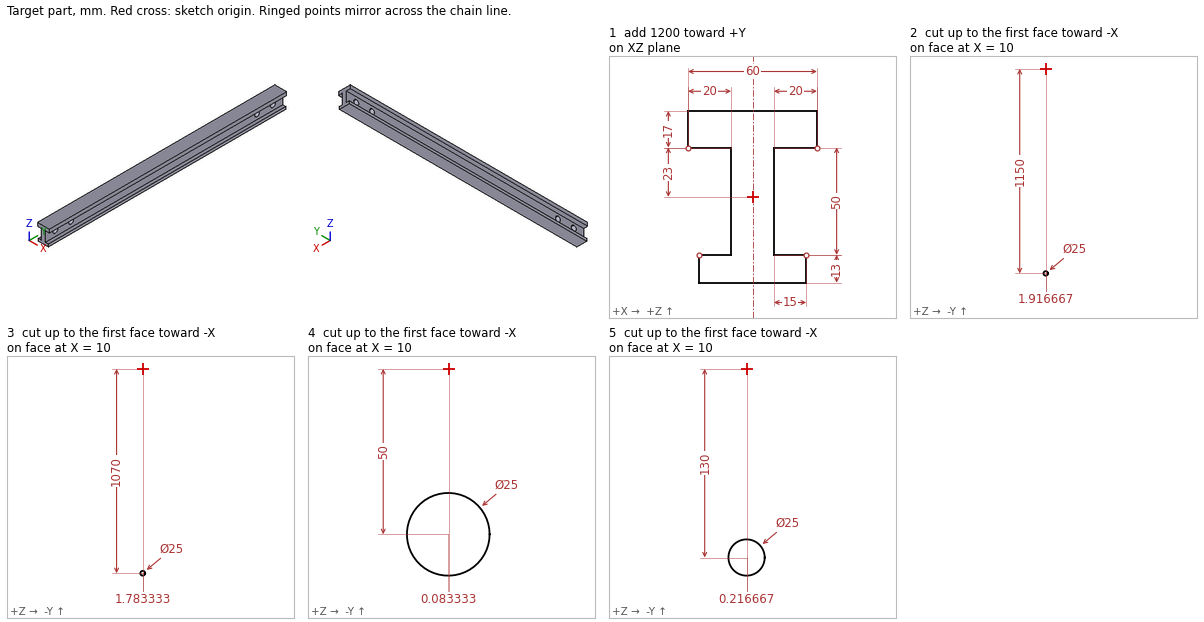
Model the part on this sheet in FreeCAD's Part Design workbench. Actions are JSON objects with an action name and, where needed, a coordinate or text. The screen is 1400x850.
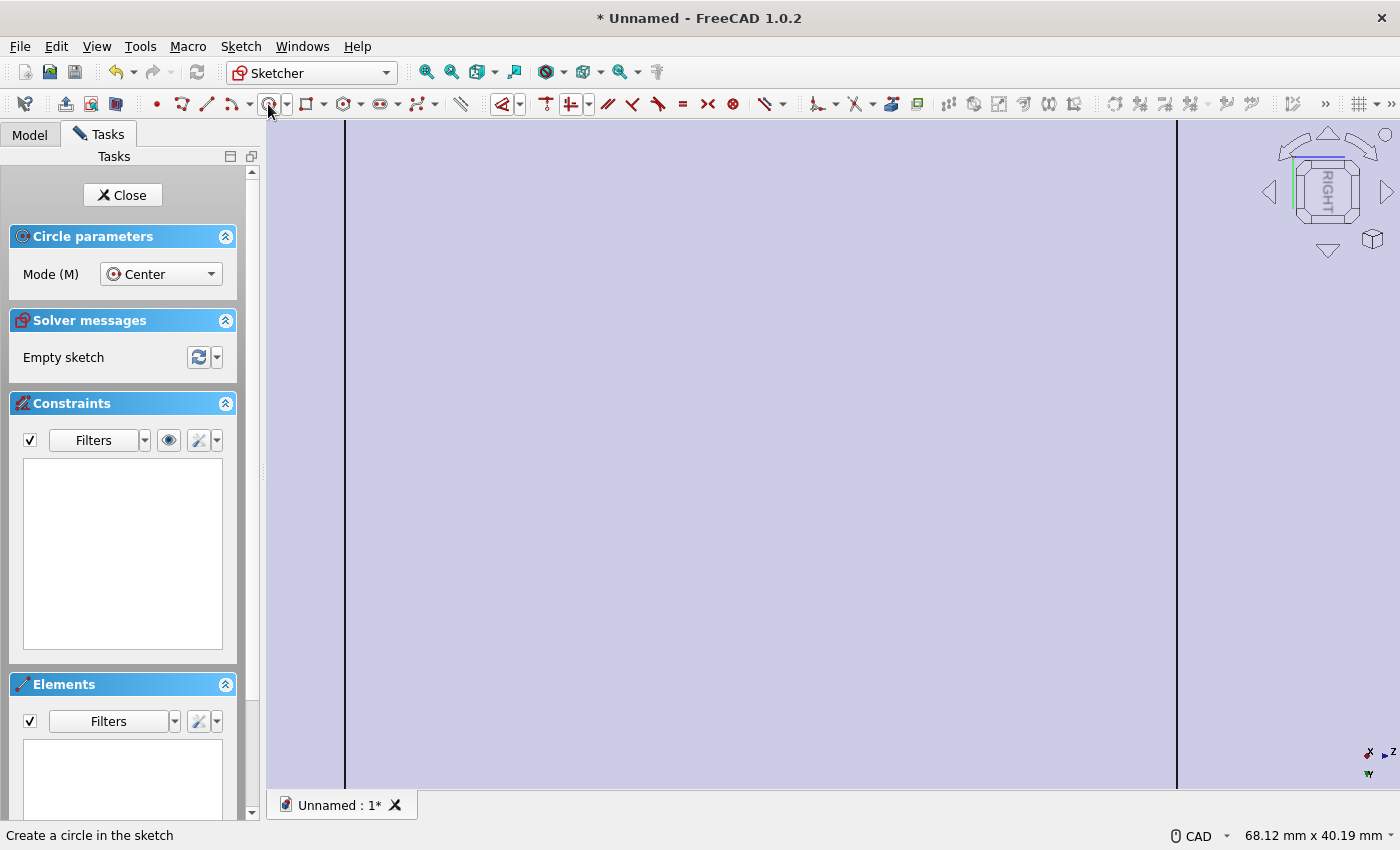
{"action": "left_click", "coordinate": [764, 454]}
{"action": "left_click", "coordinate": [912, 307]}
{"action": "key", "text": "Escape"}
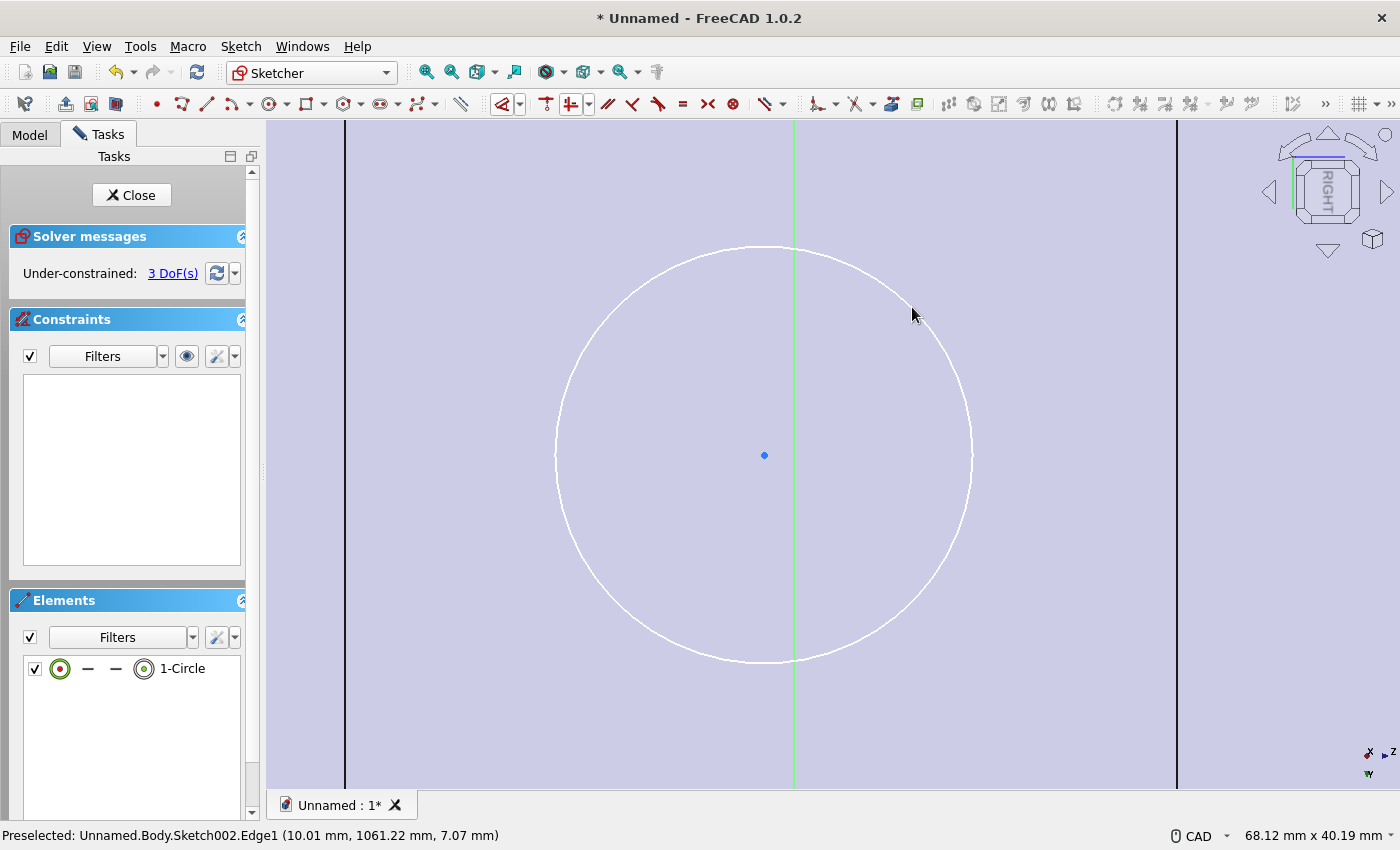
{"action": "left_click", "coordinate": [911, 307]}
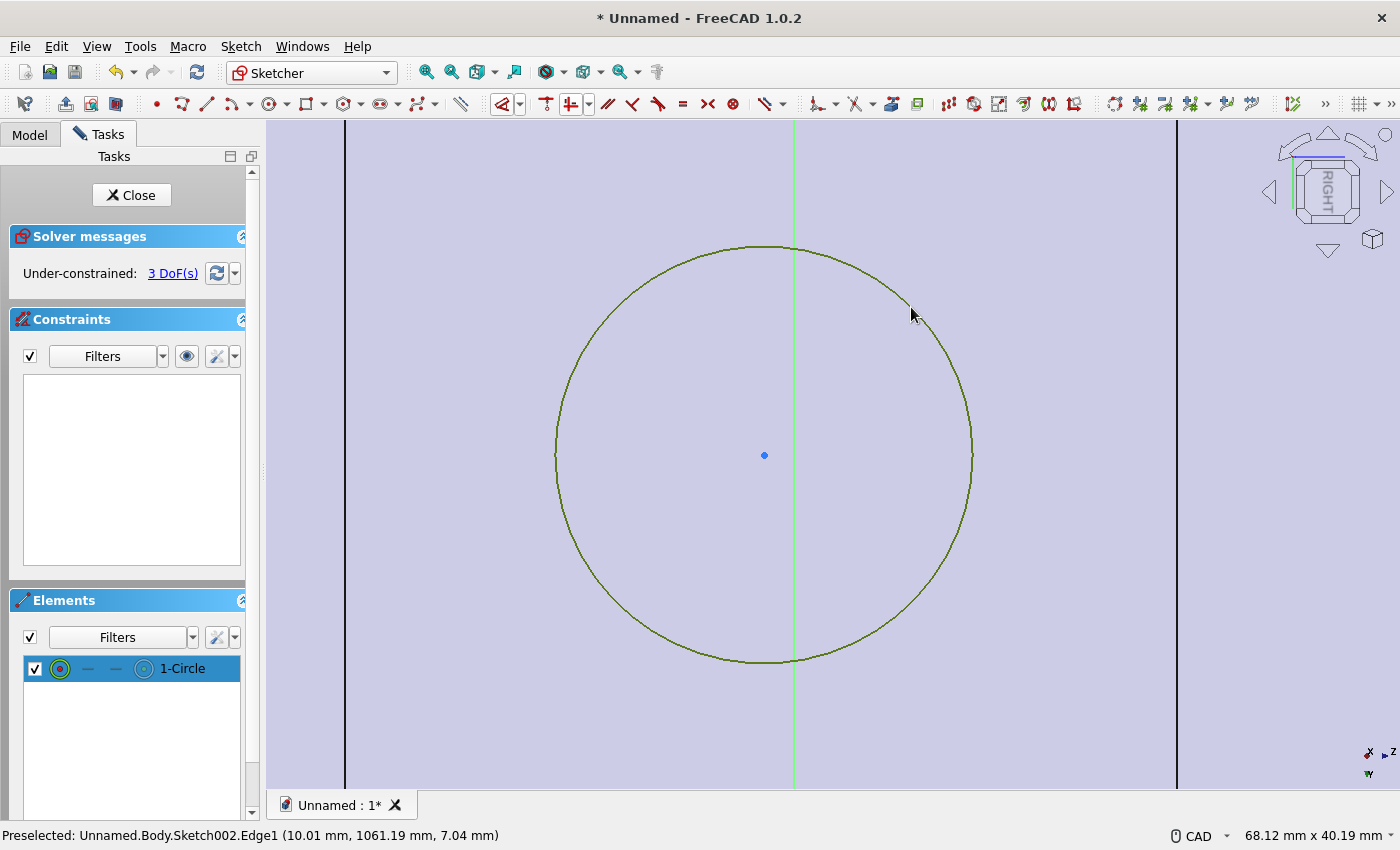
{"action": "left_click", "coordinate": [520, 104]}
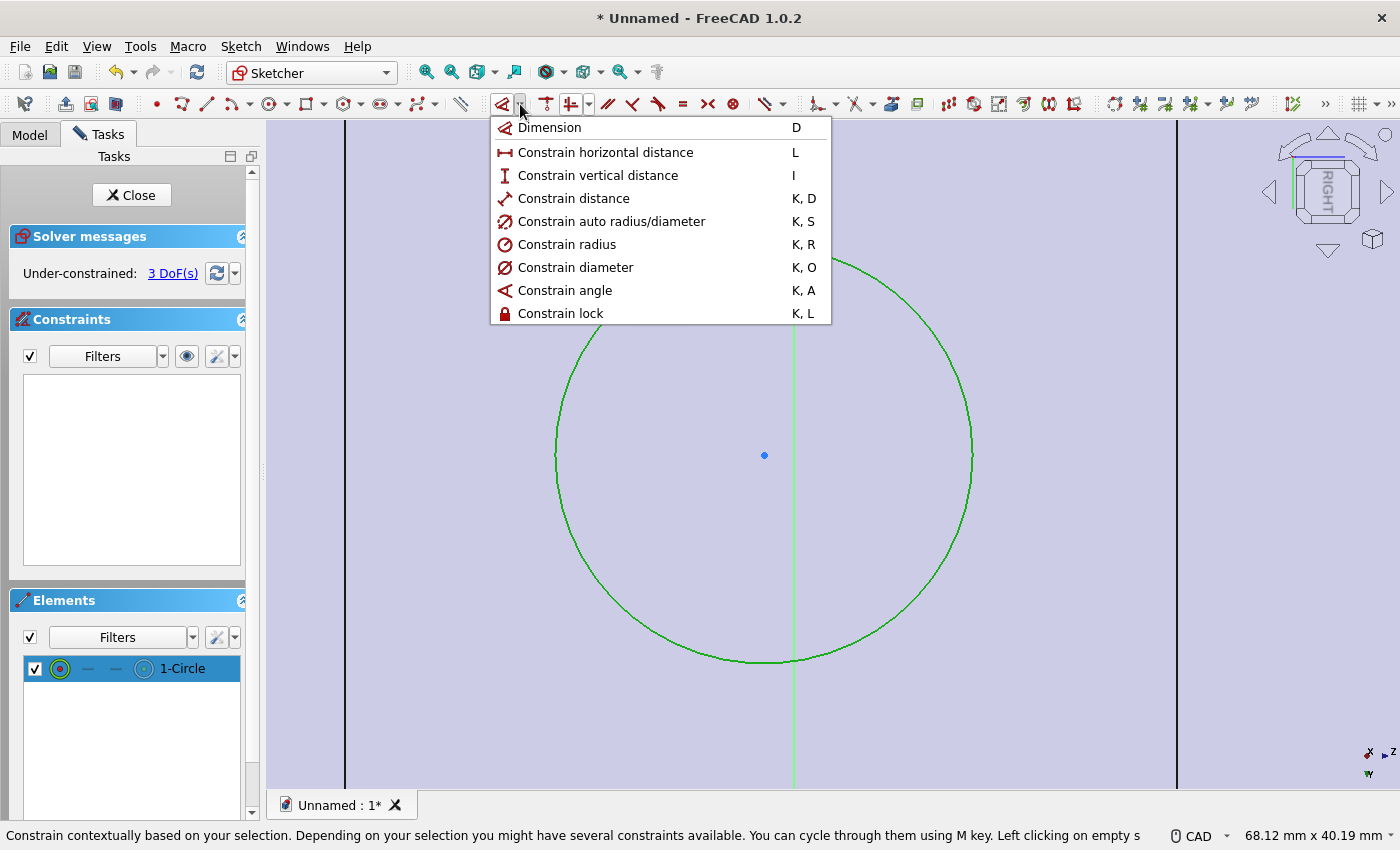
{"action": "left_click", "coordinate": [661, 268]}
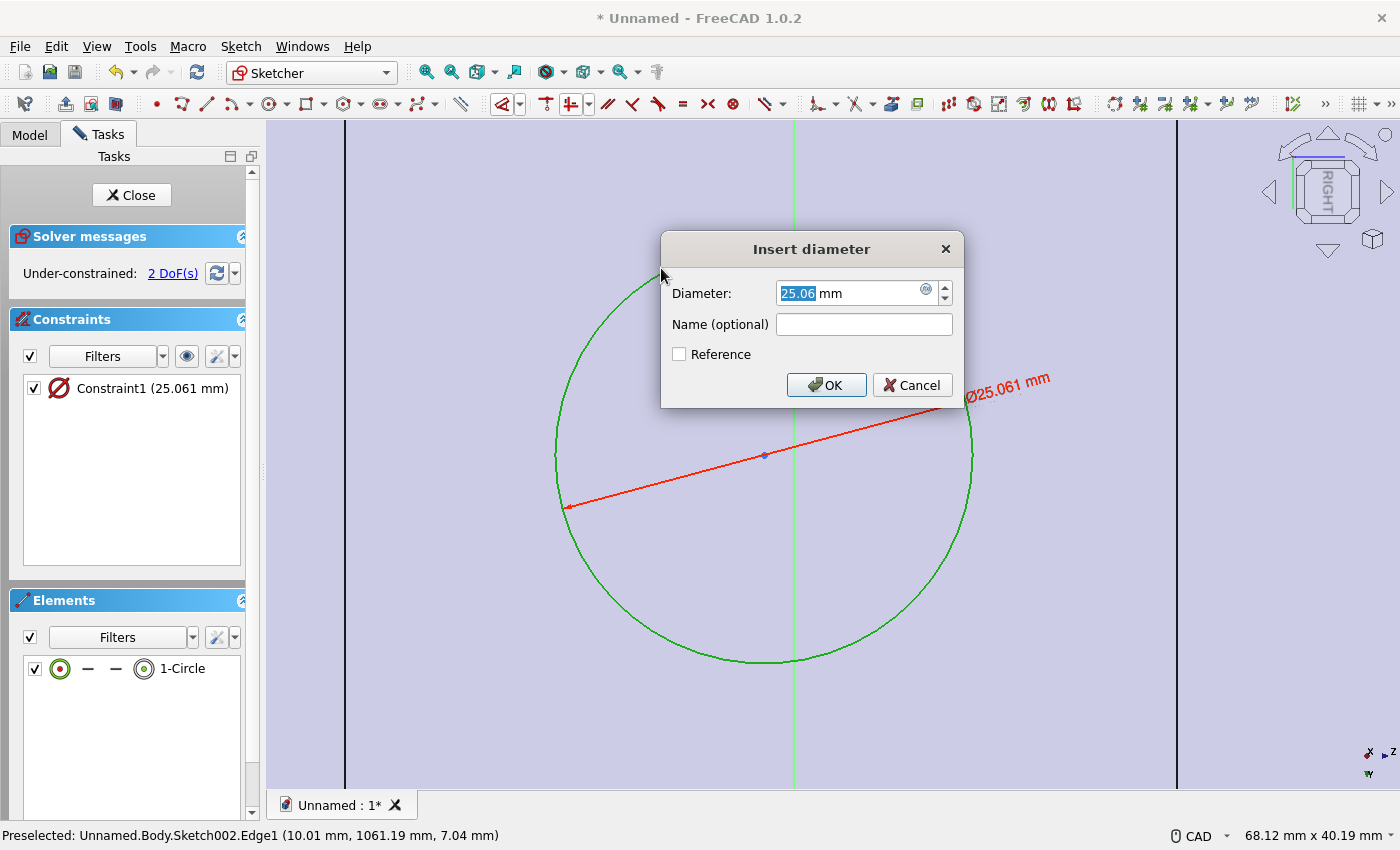
{"action": "type", "text": "25"}
{"action": "key", "text": "Return"}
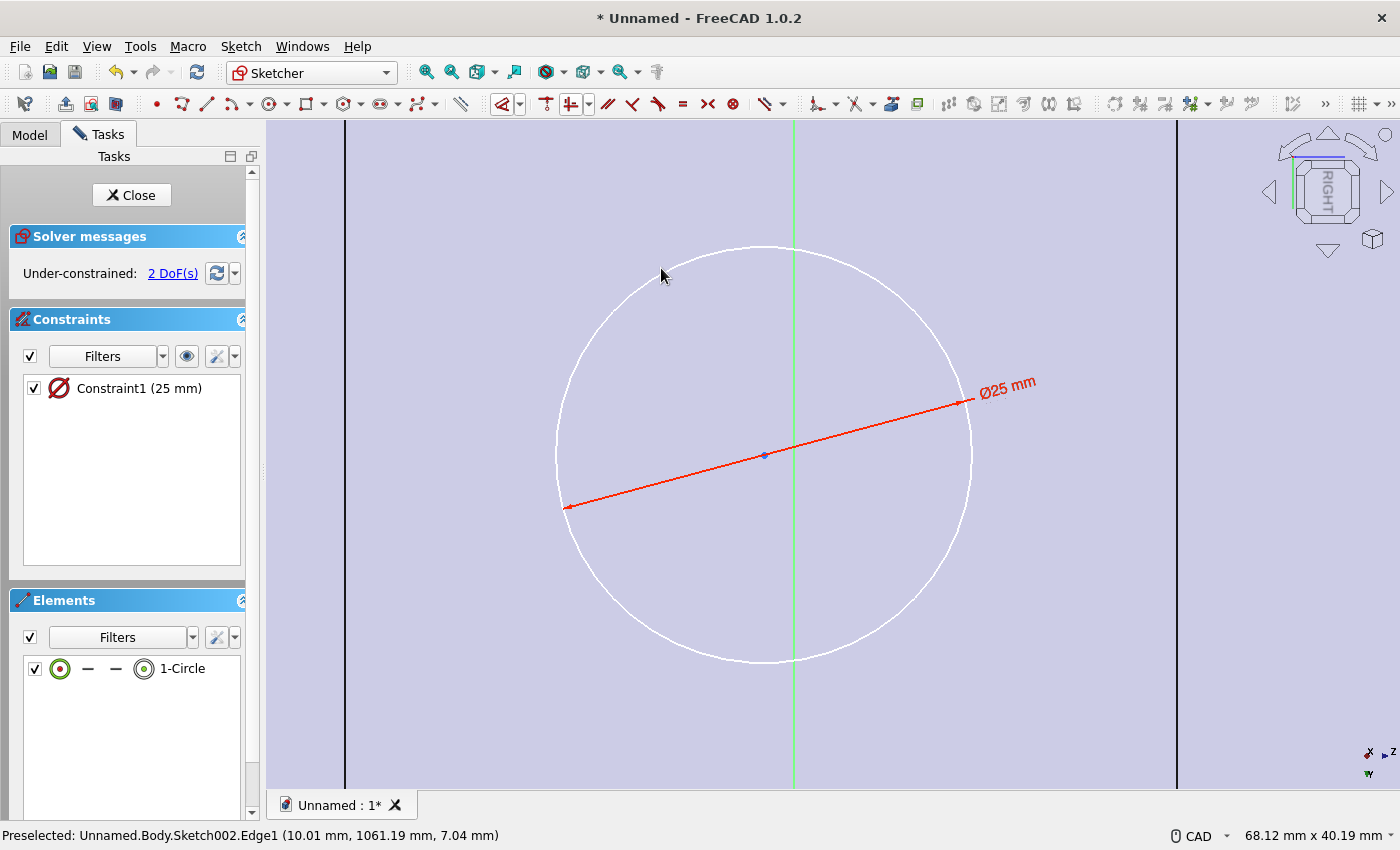
{"action": "left_click", "coordinate": [764, 455]}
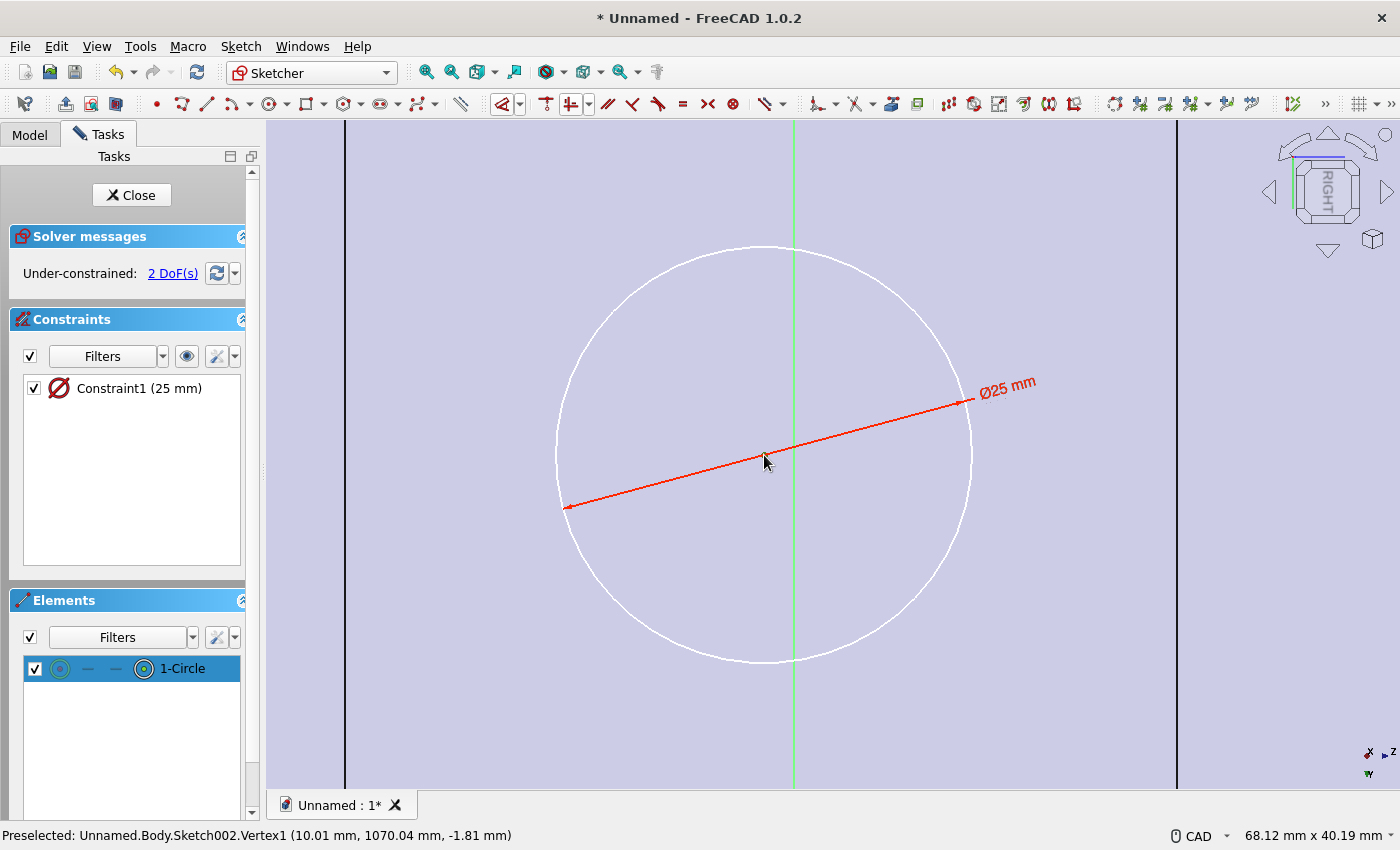
{"action": "left_click", "coordinate": [520, 104]}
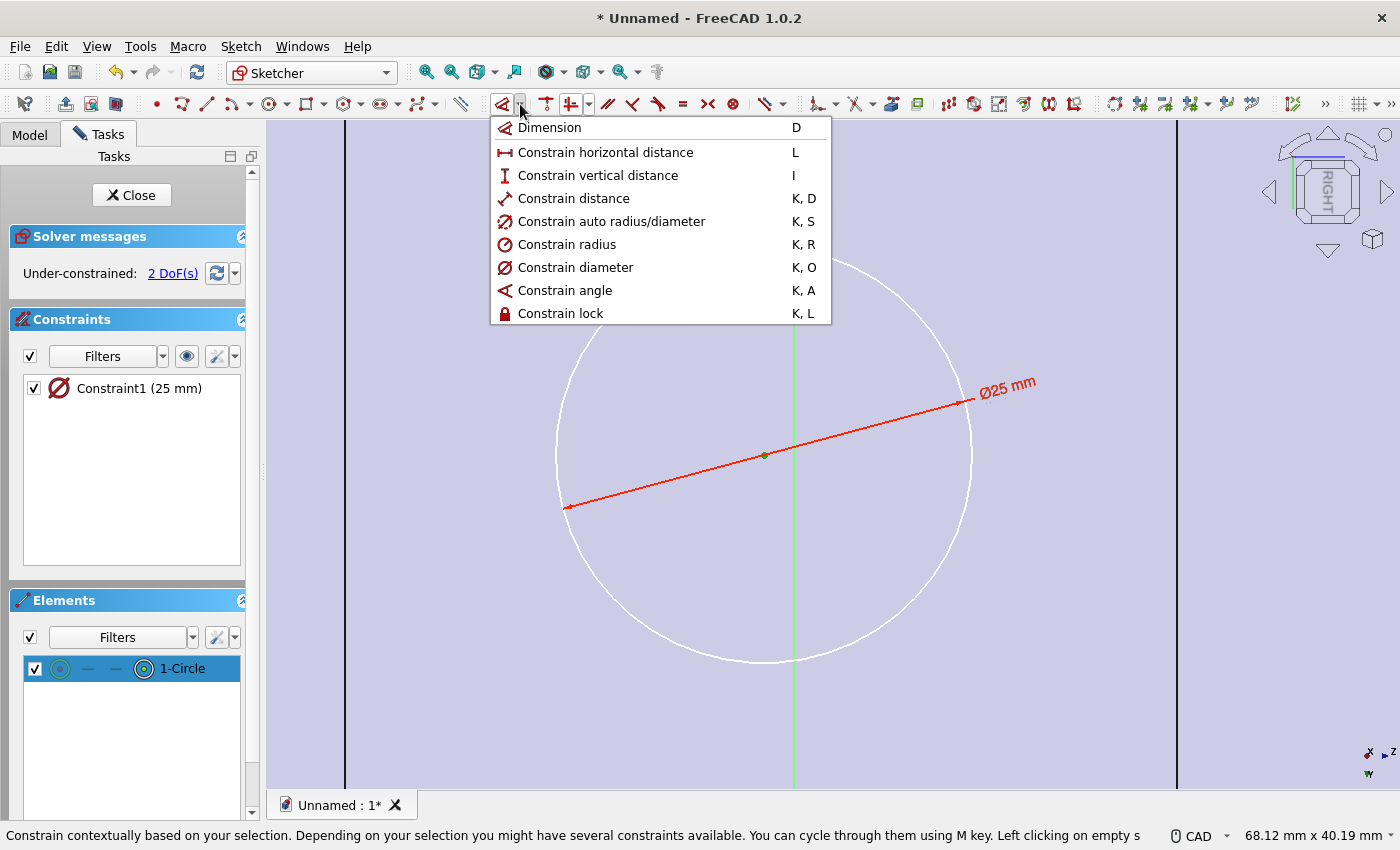
{"action": "left_click", "coordinate": [661, 176]}